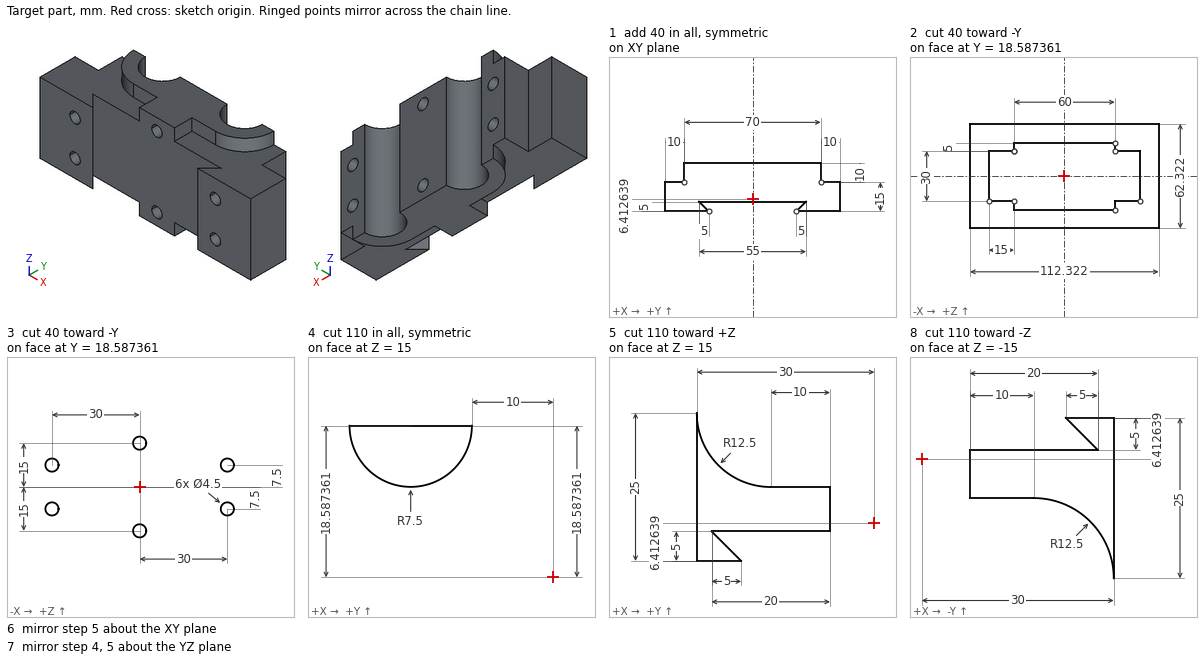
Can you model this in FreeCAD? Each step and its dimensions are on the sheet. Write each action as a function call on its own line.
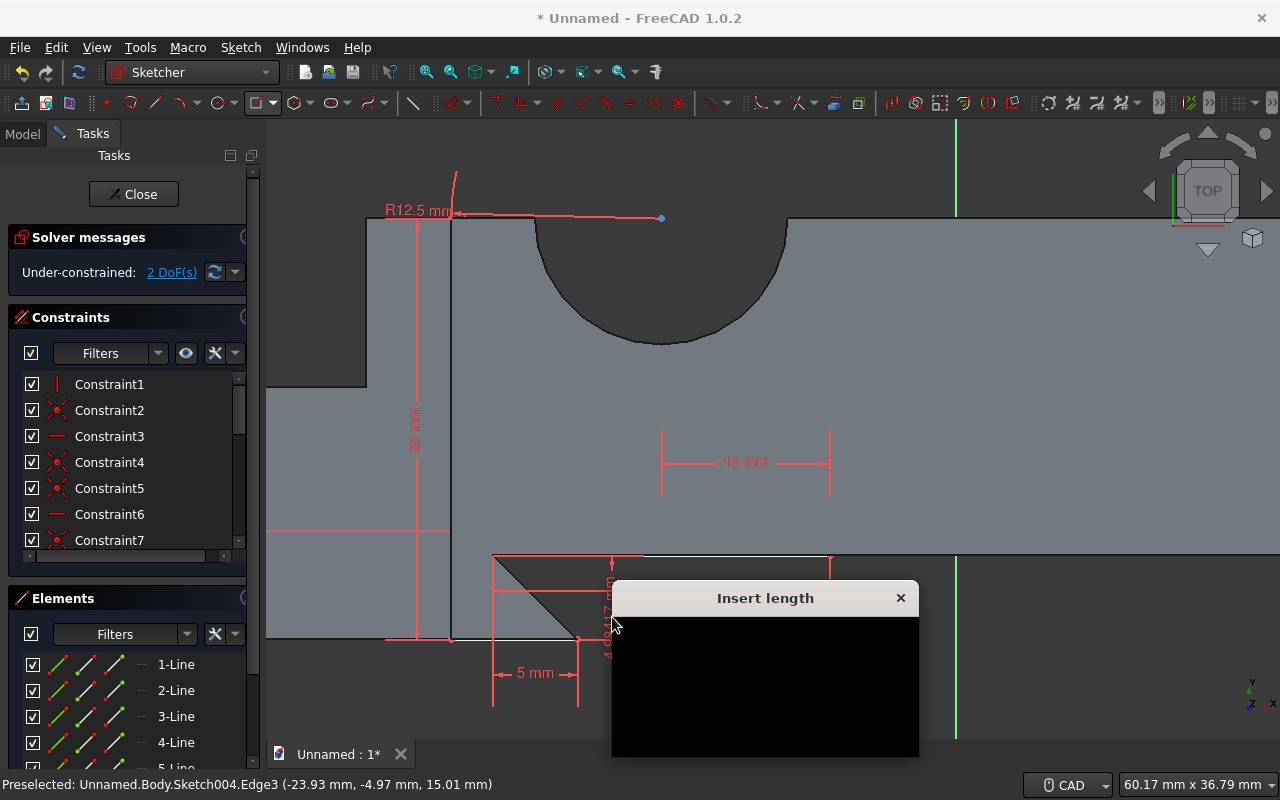
text(5)
key(Return)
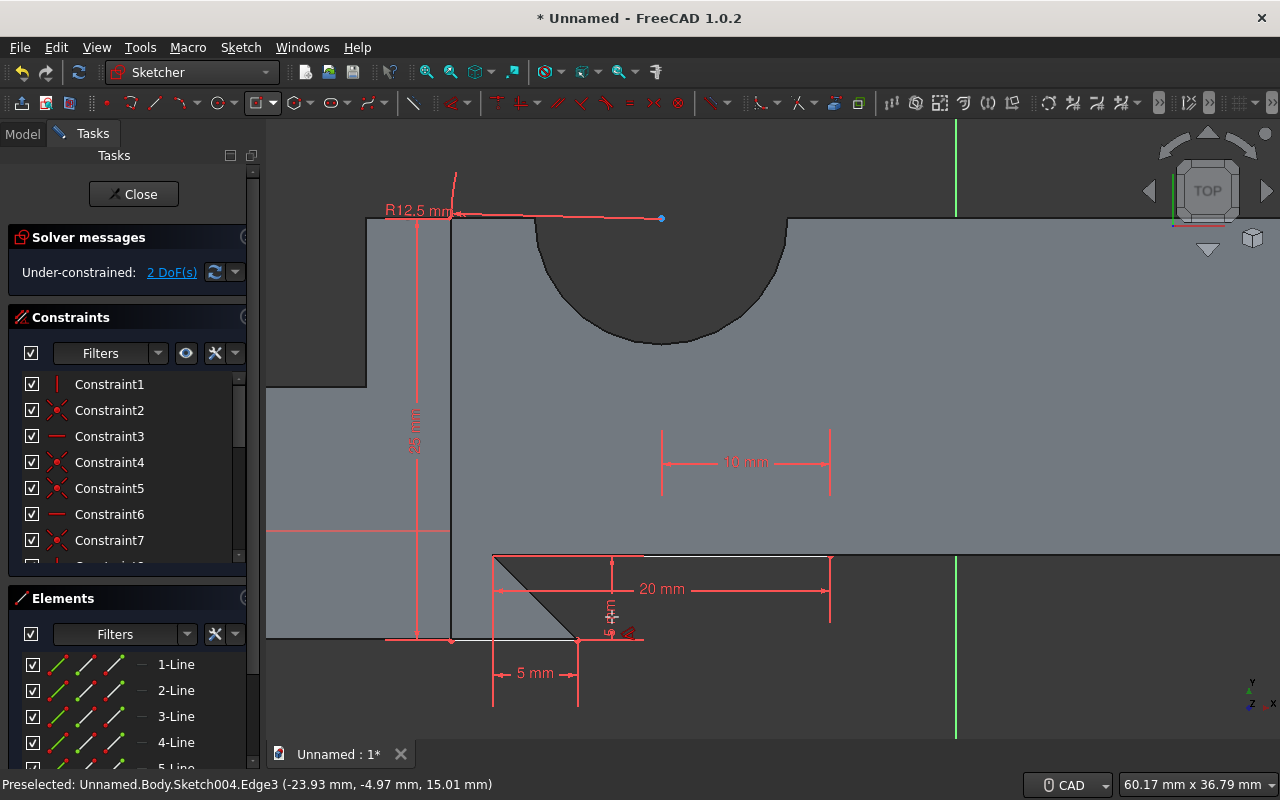
click(451, 219)
click(704, 185)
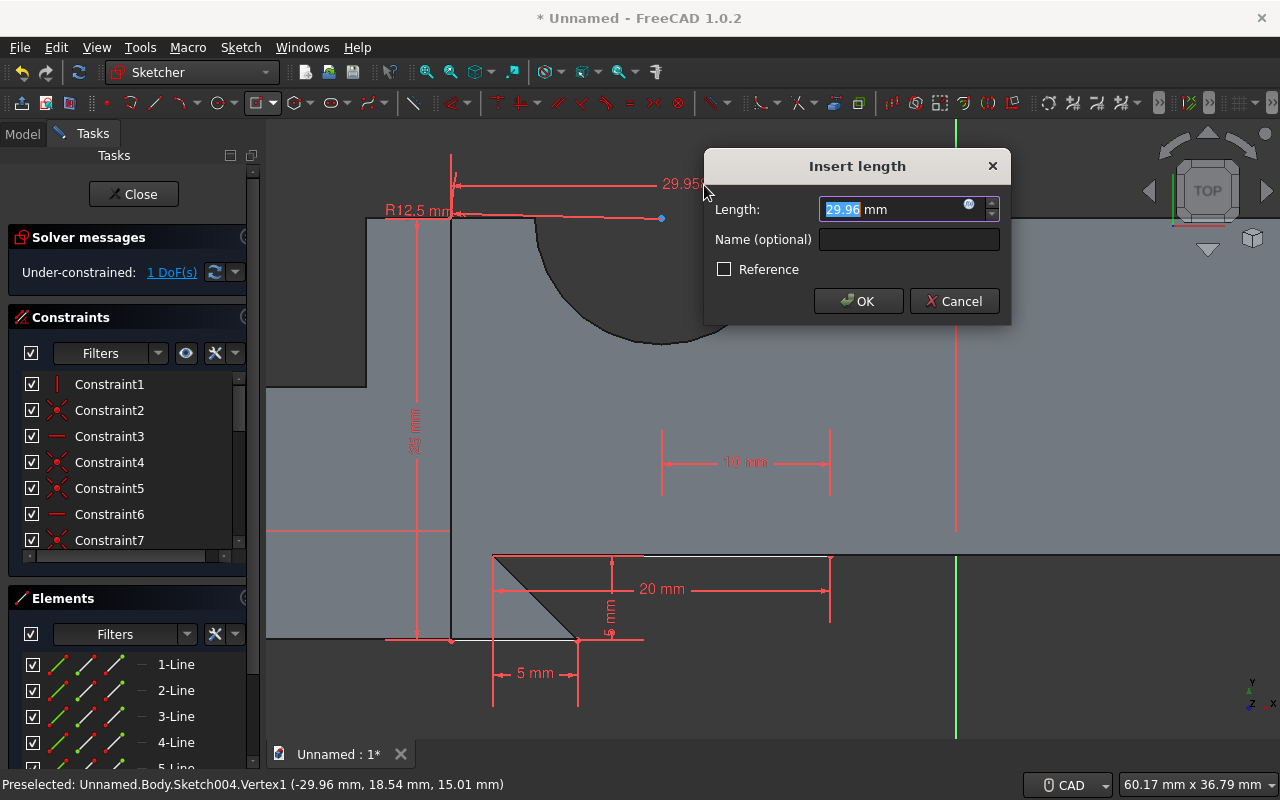
text(30)
key(Return)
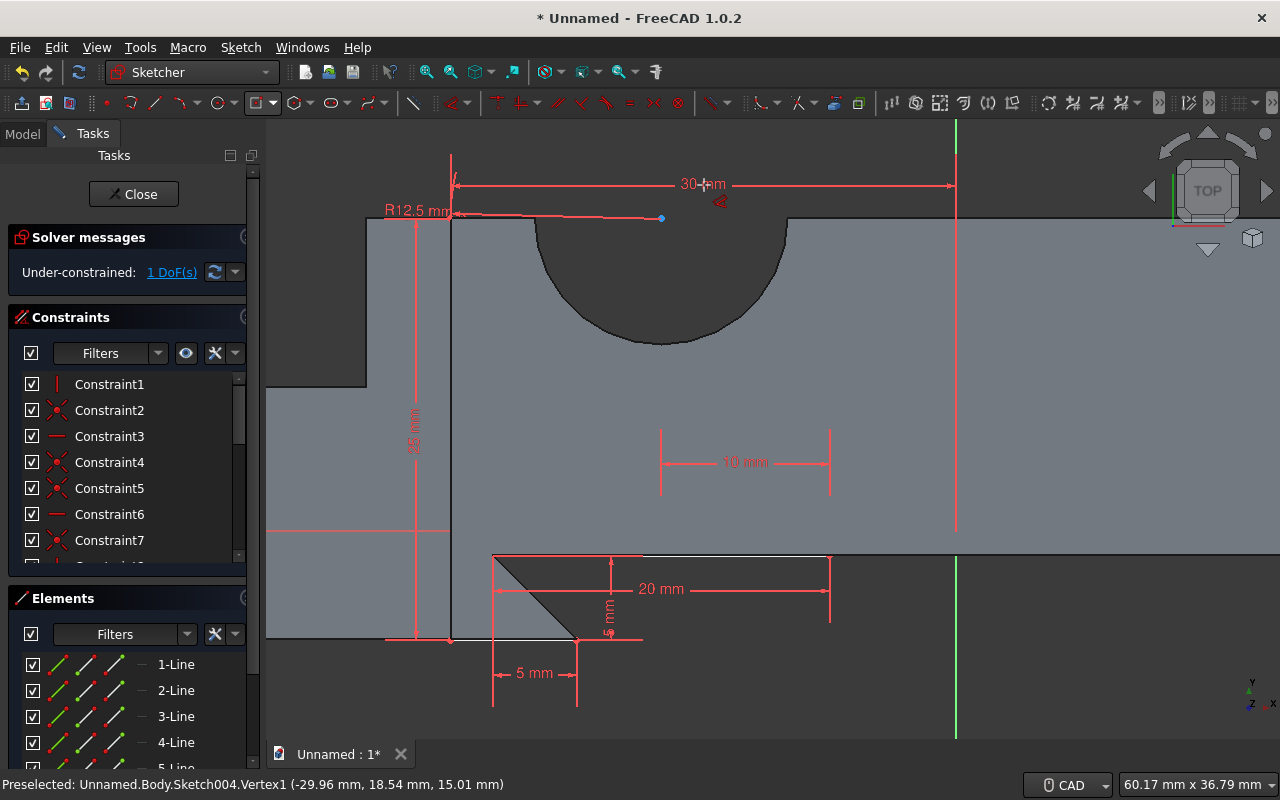
click(451, 640)
click(990, 586)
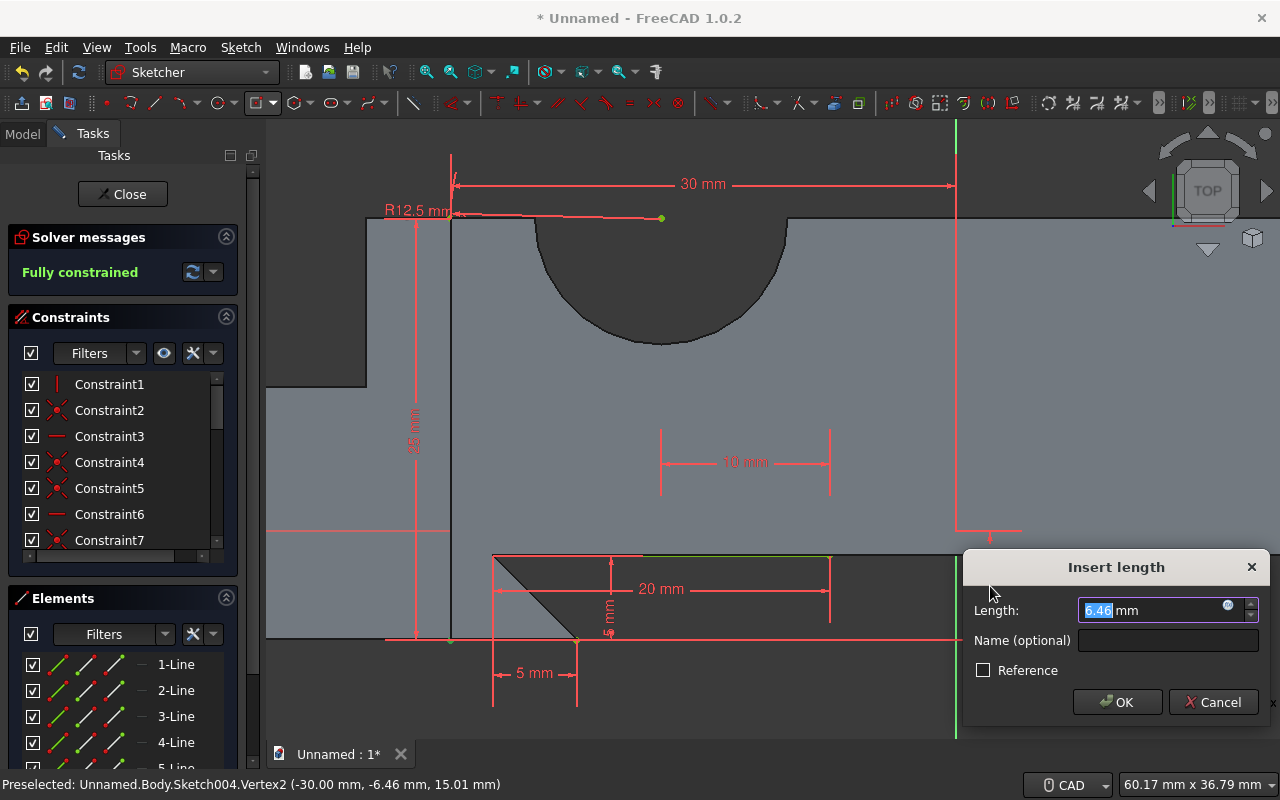
text(6.412639)
key(Return)
key(Escape)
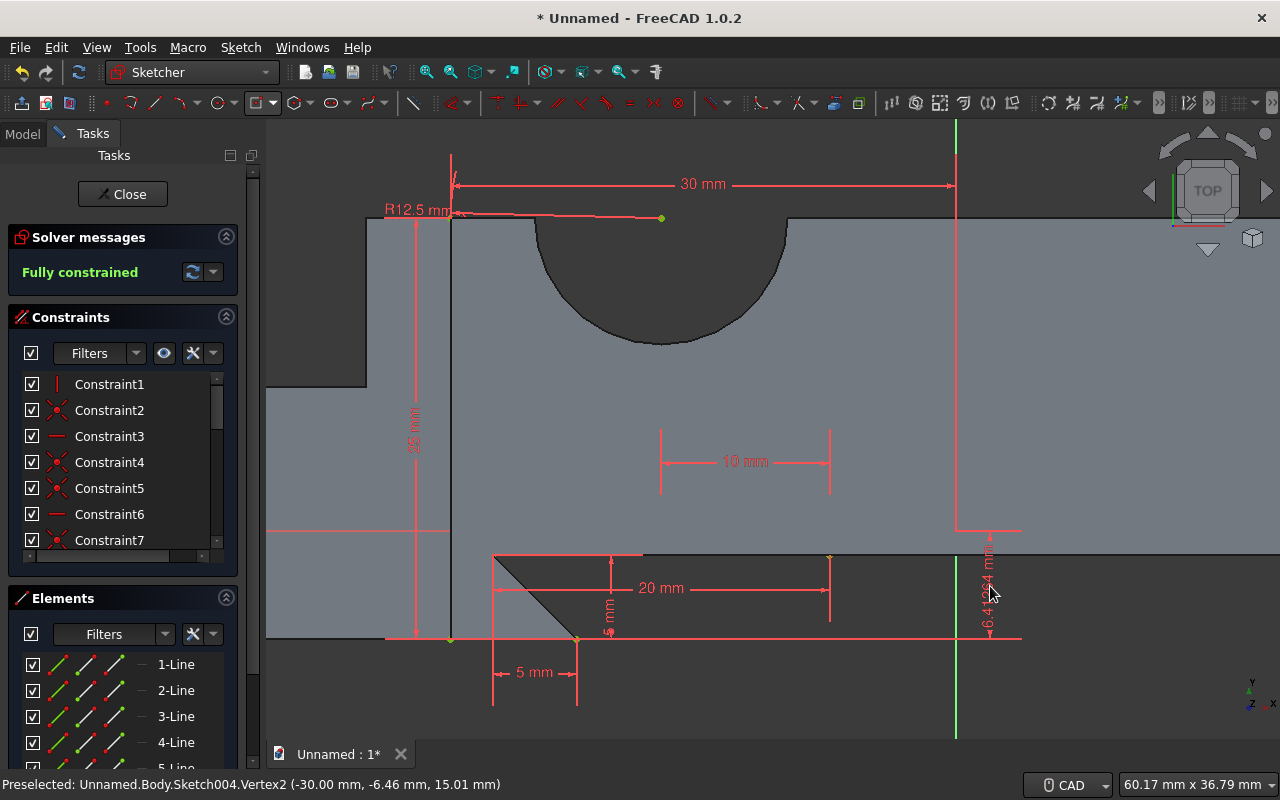
click(123, 194)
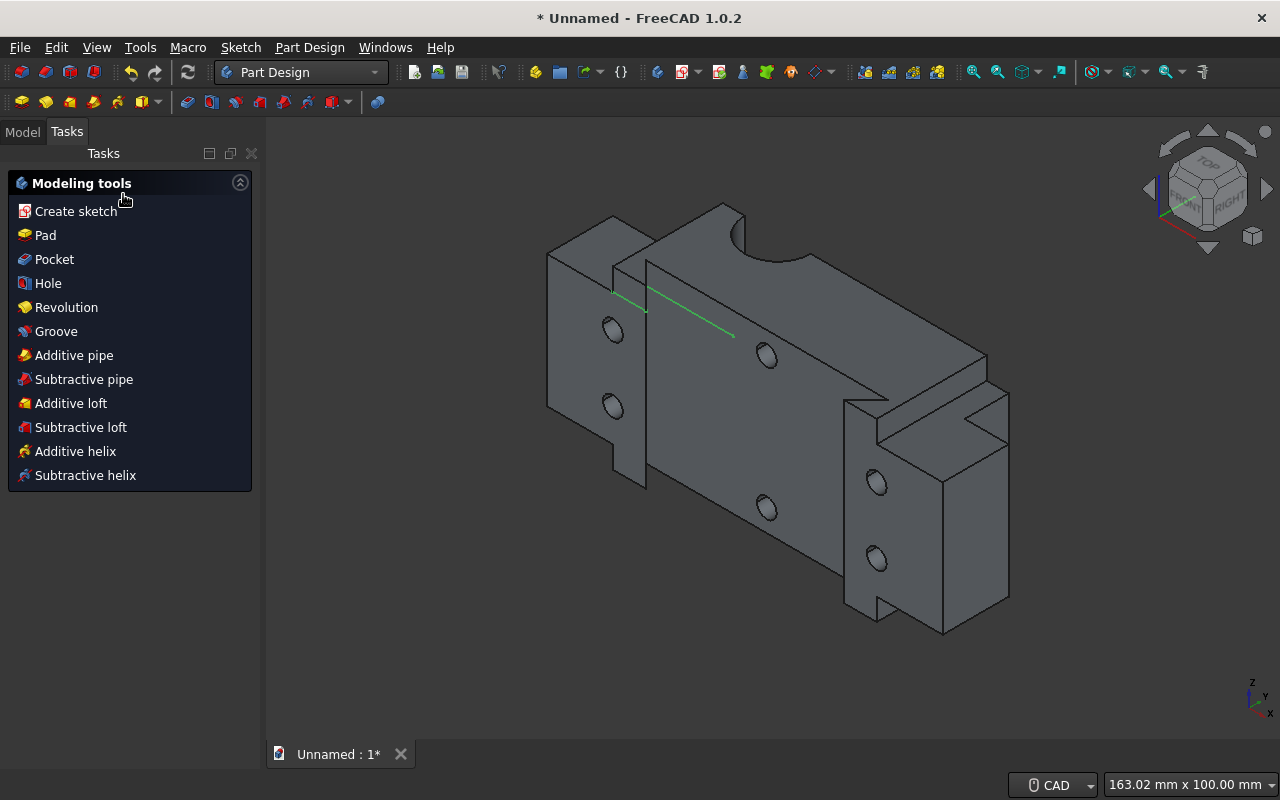
click(188, 102)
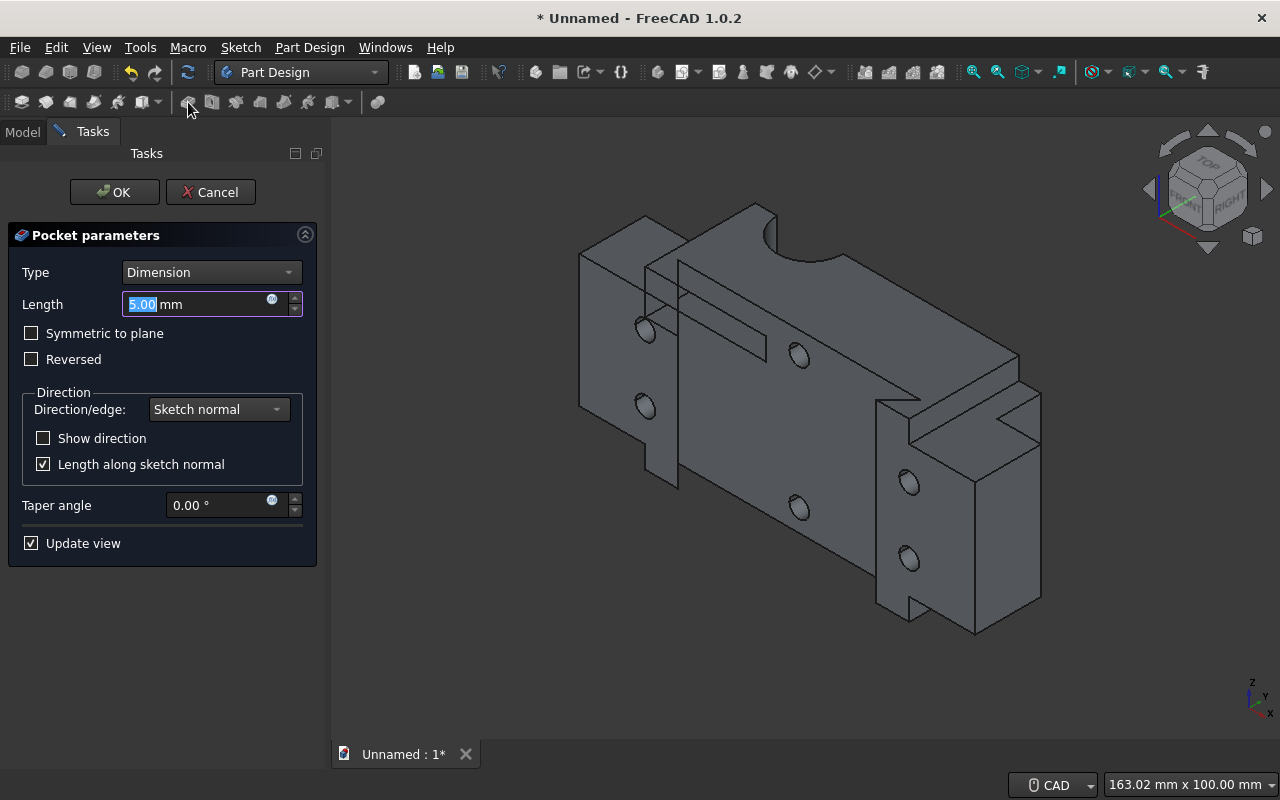
text(110)
key(Tab)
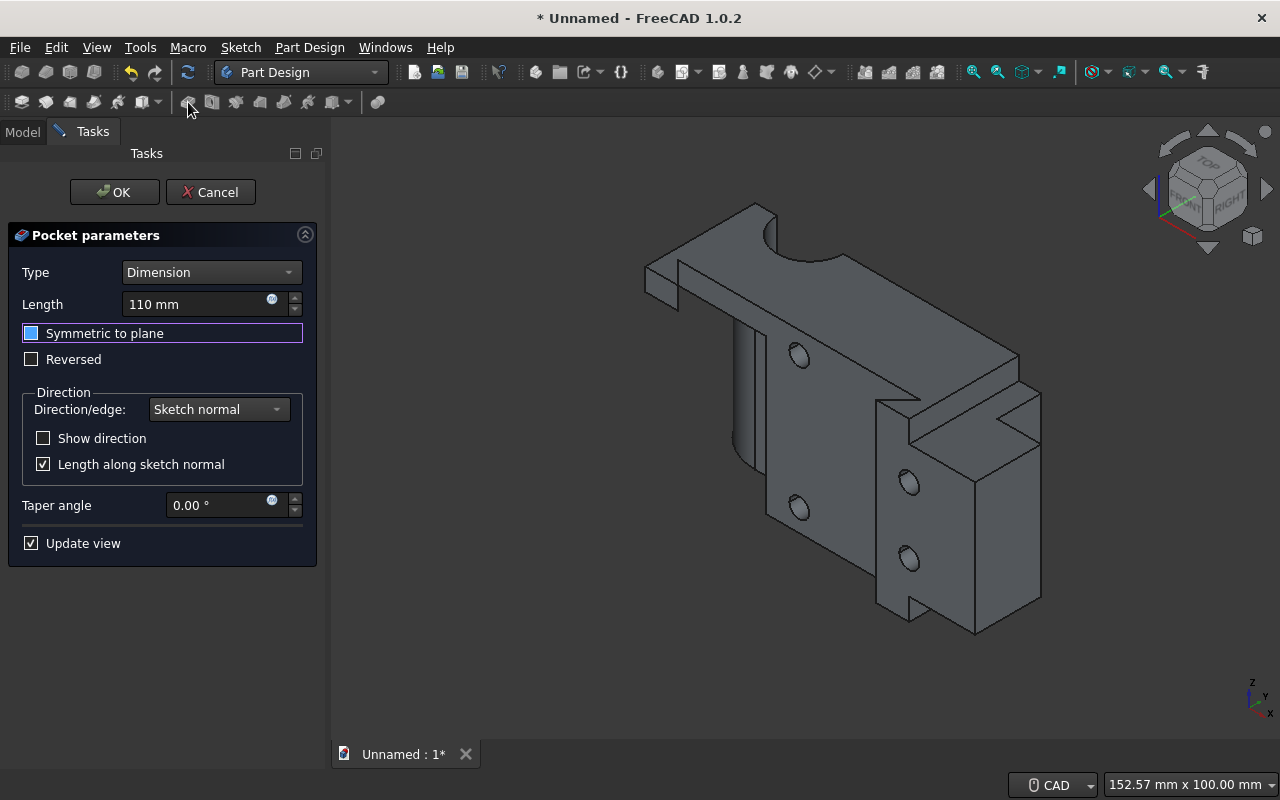
click(30, 359)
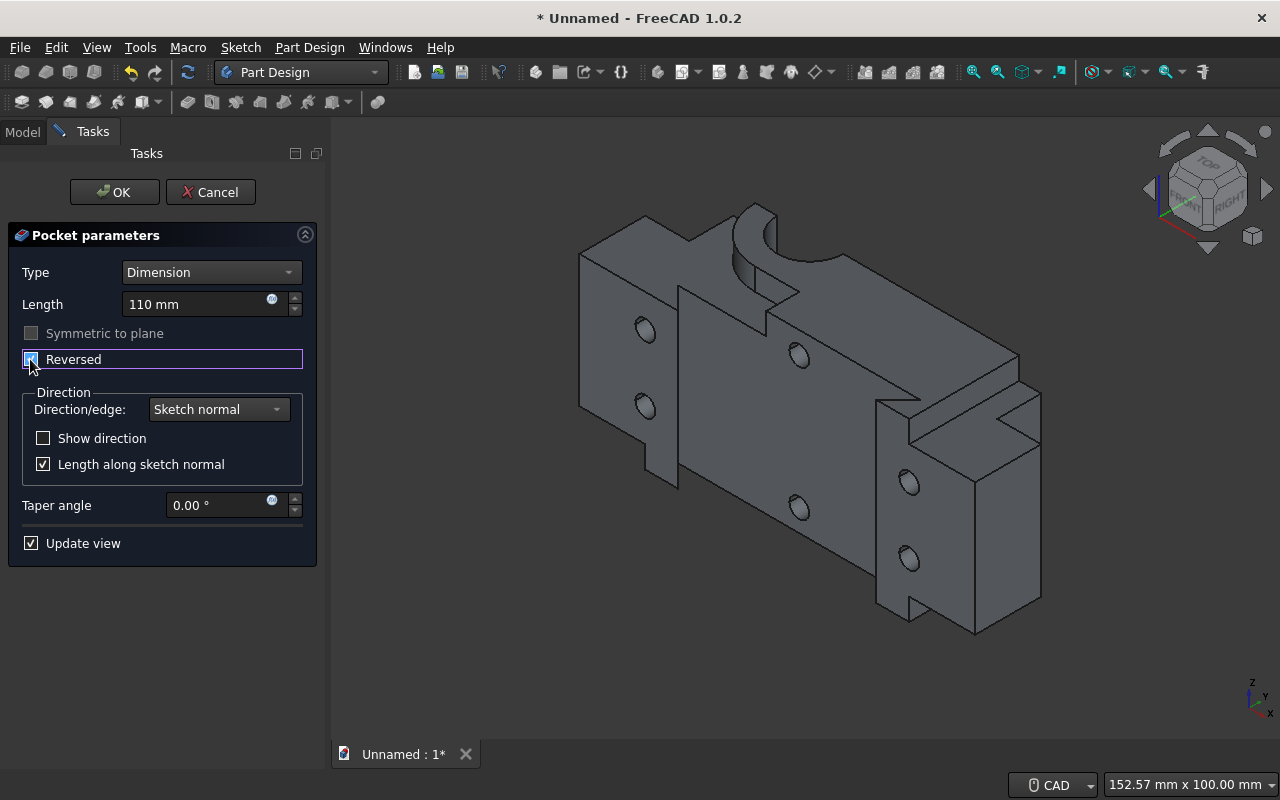
click(115, 192)